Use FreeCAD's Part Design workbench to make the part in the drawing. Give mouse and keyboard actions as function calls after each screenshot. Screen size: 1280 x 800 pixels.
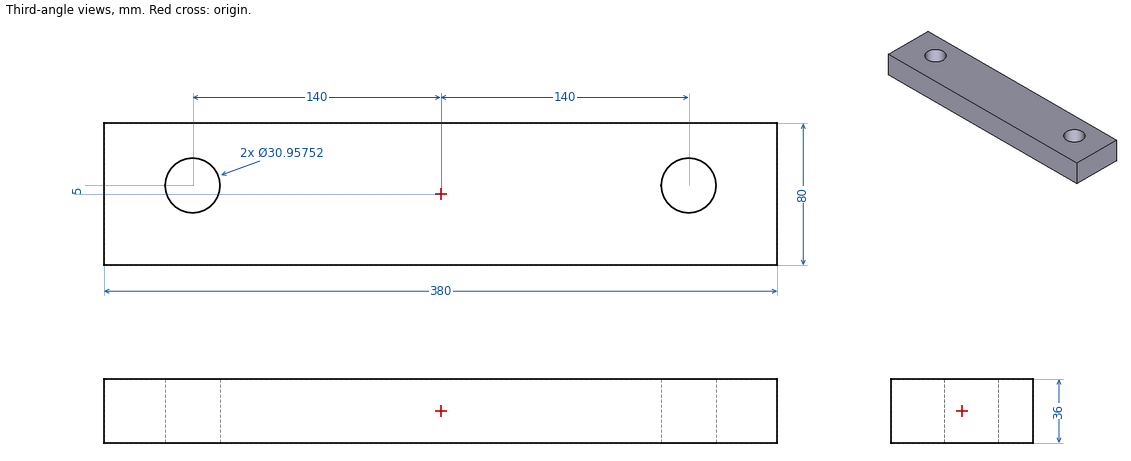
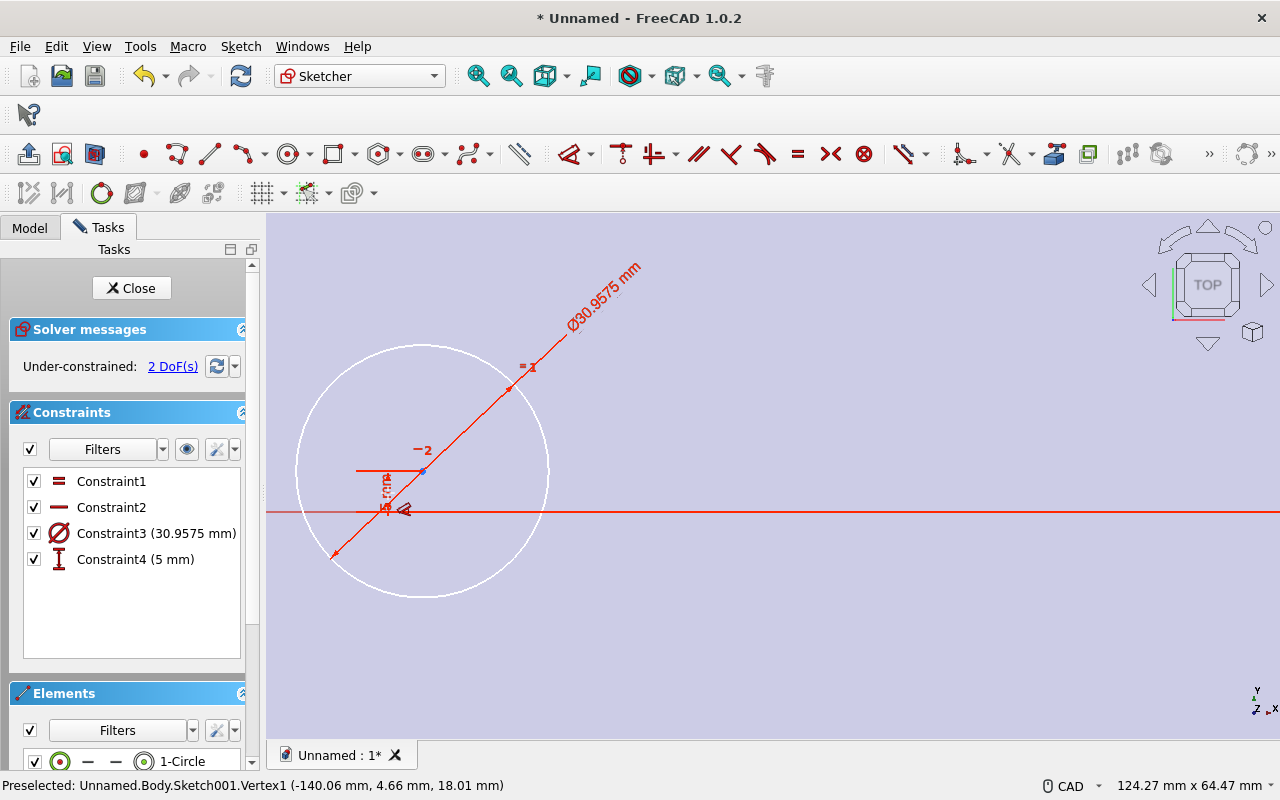
scroll(423, 478, down, 7)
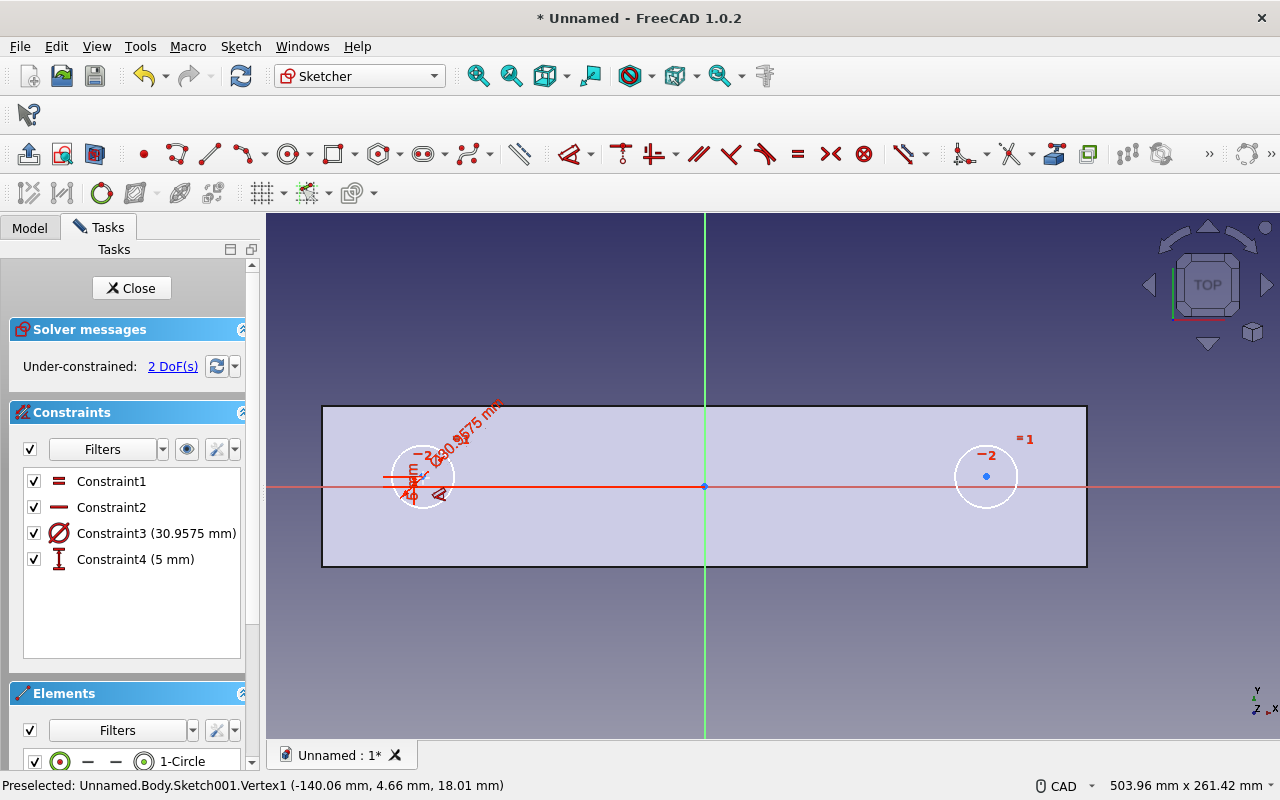
click(423, 477)
click(564, 521)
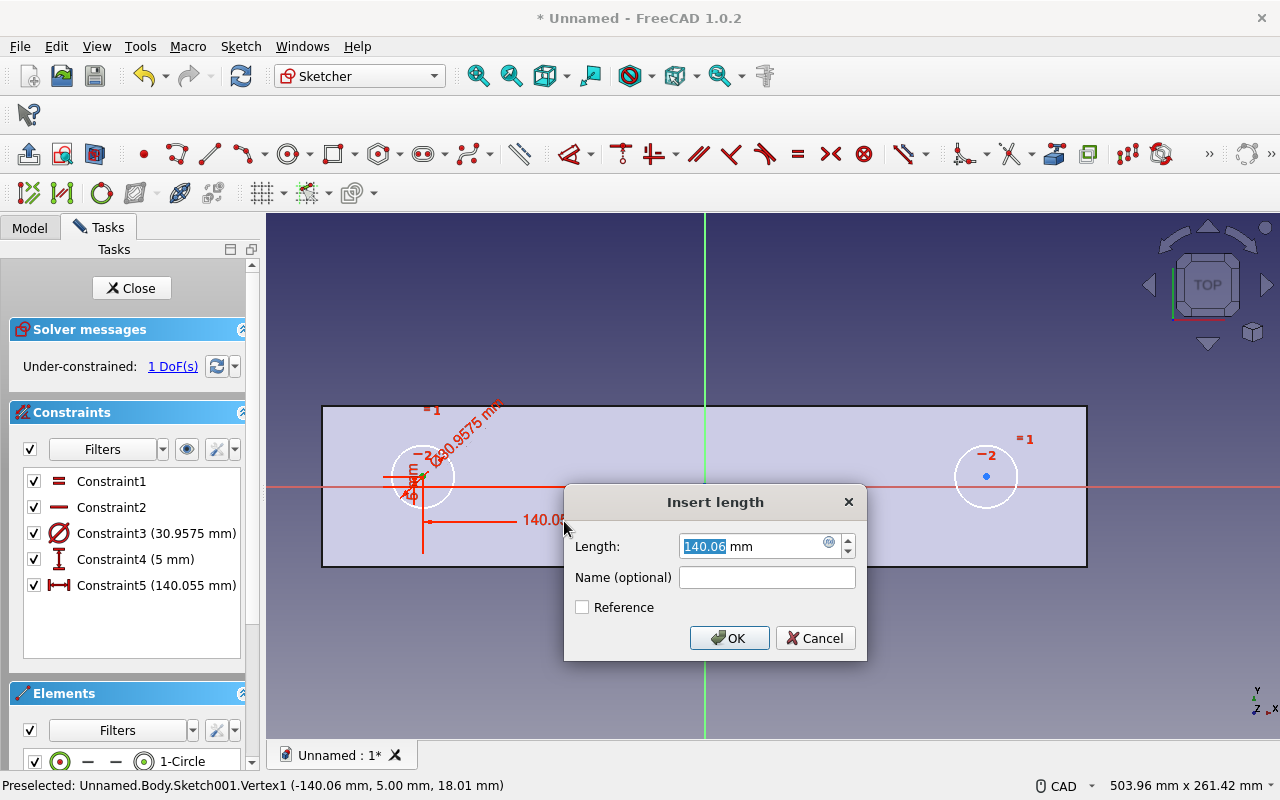
text(140)
key(Return)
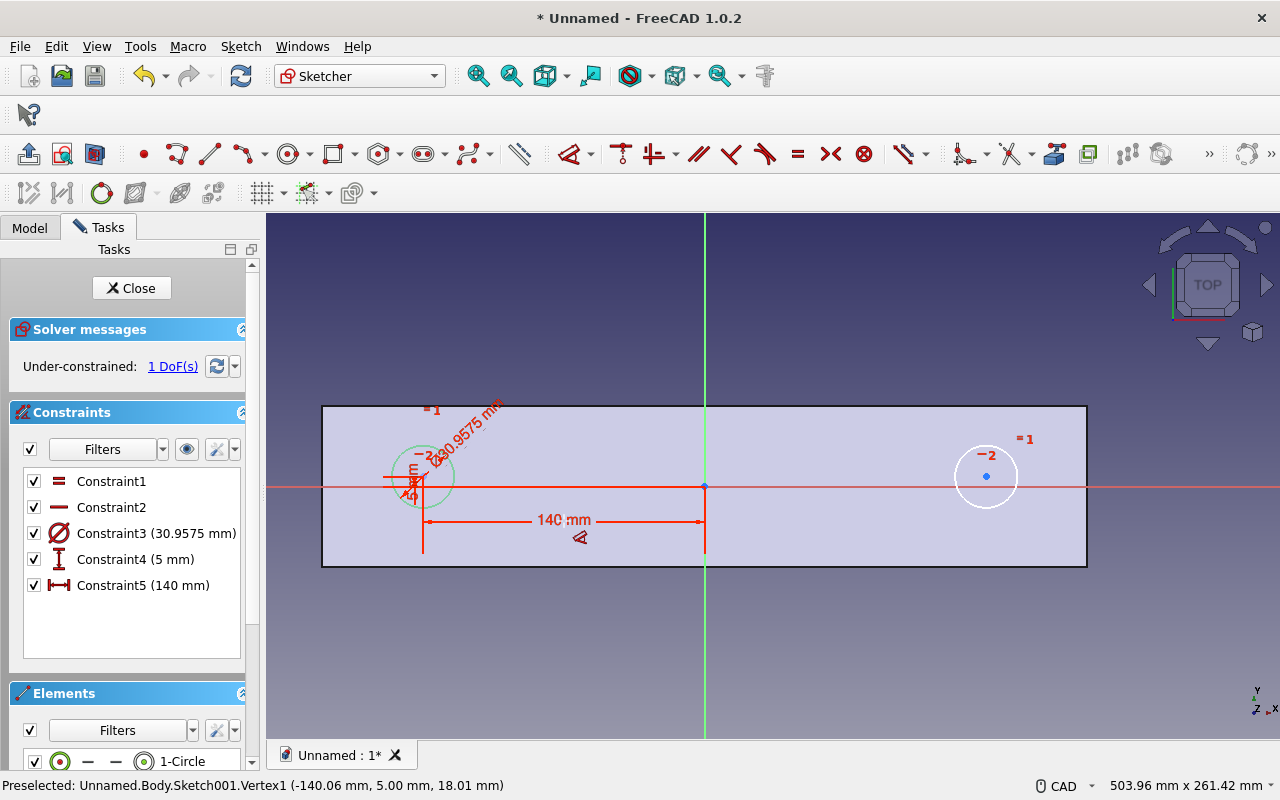
click(986, 477)
click(846, 521)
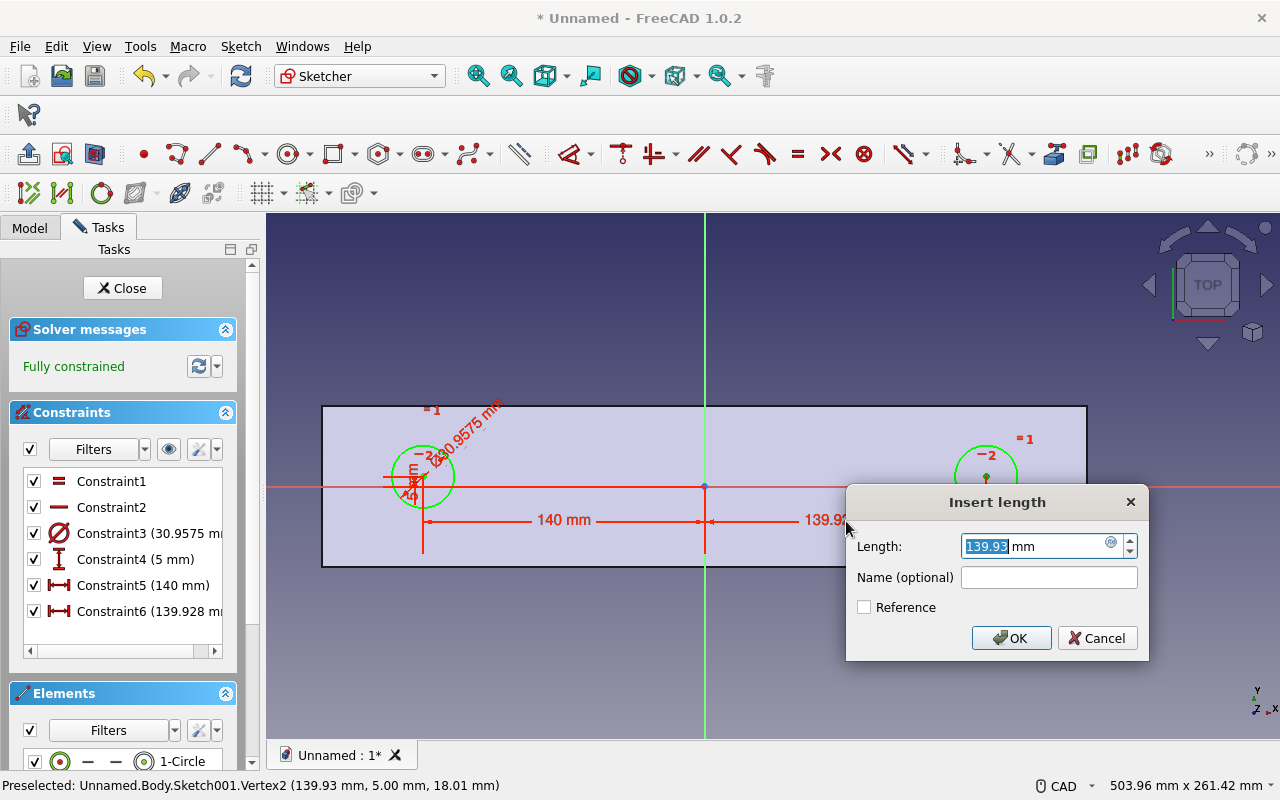
text(140)
key(Return)
key(Escape)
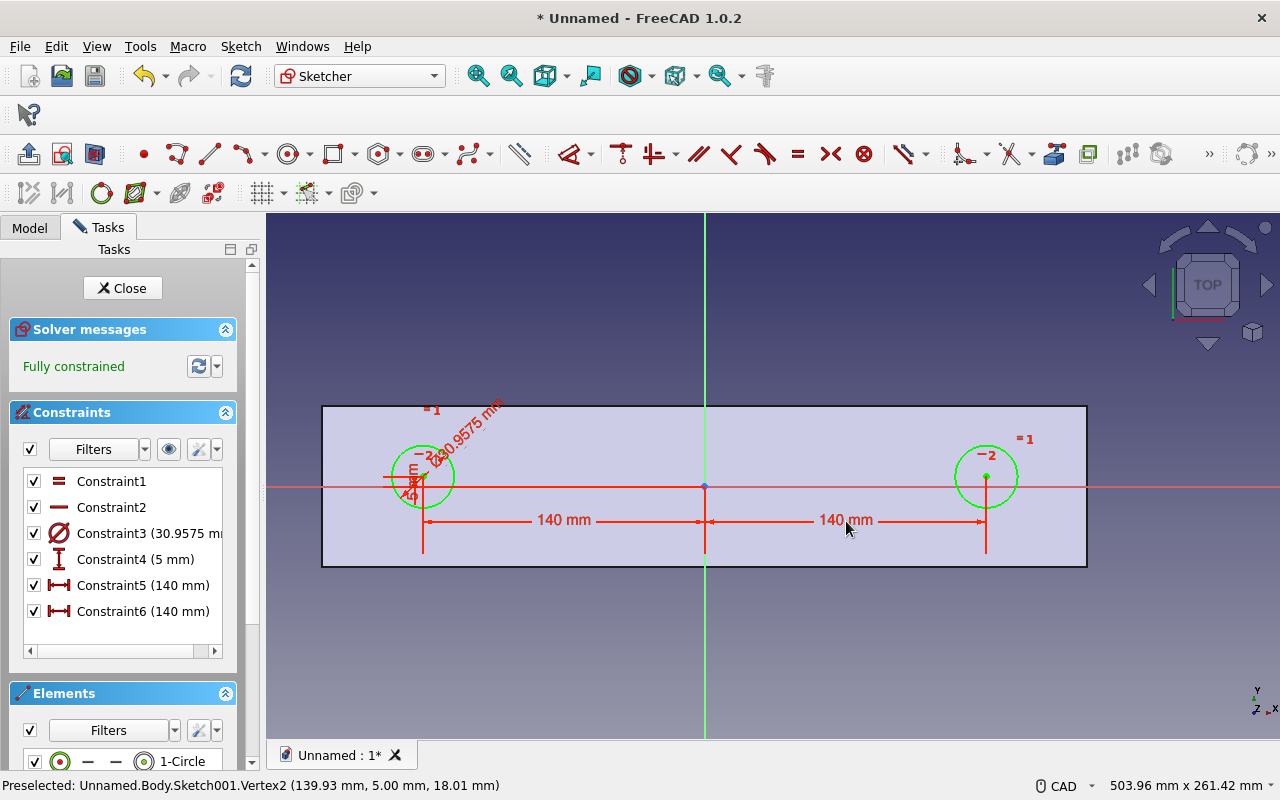
click(123, 288)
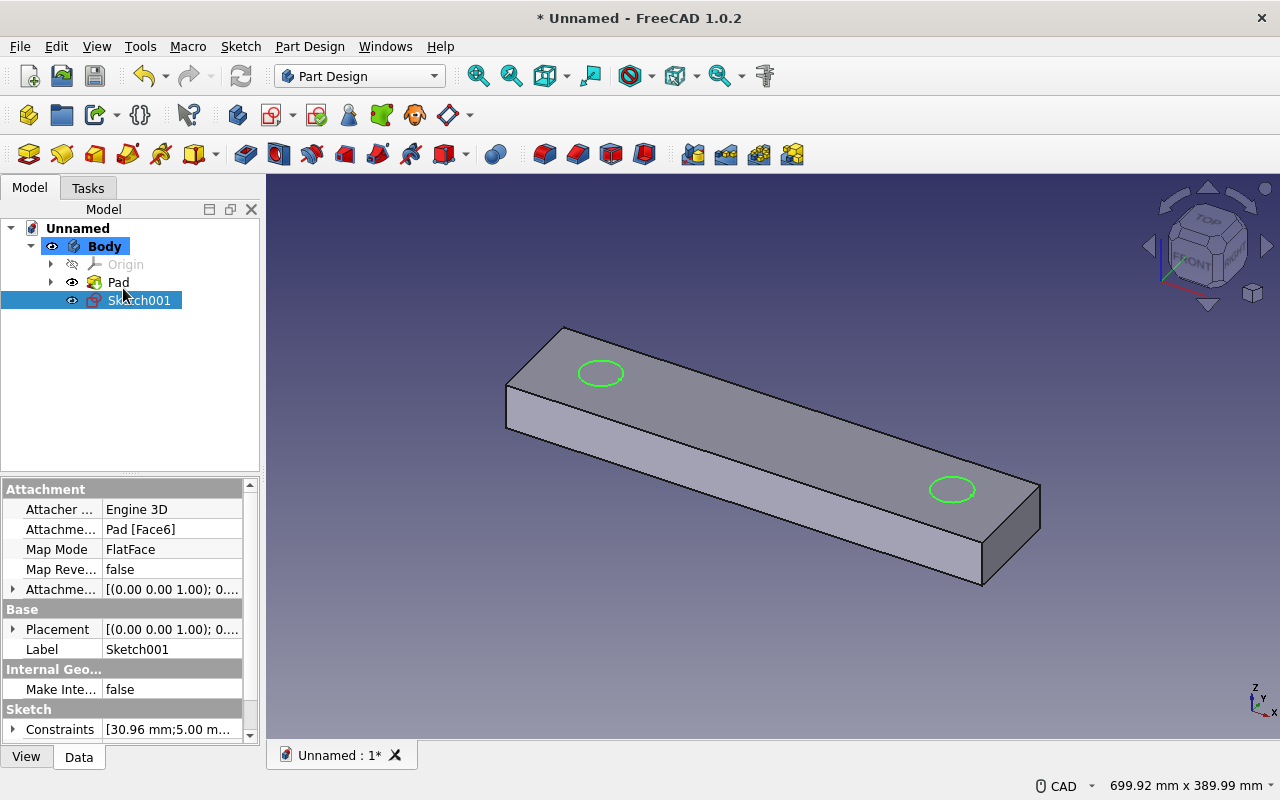
click(246, 154)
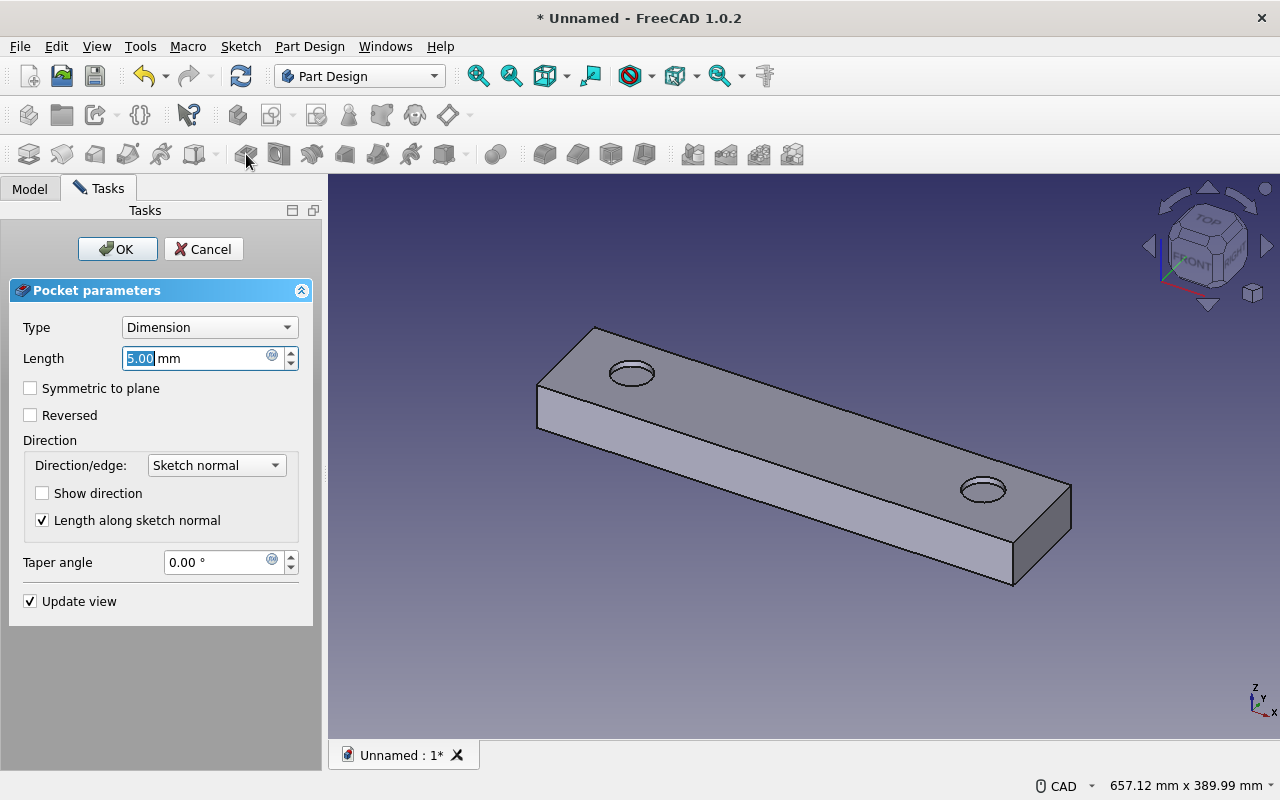
click(210, 328)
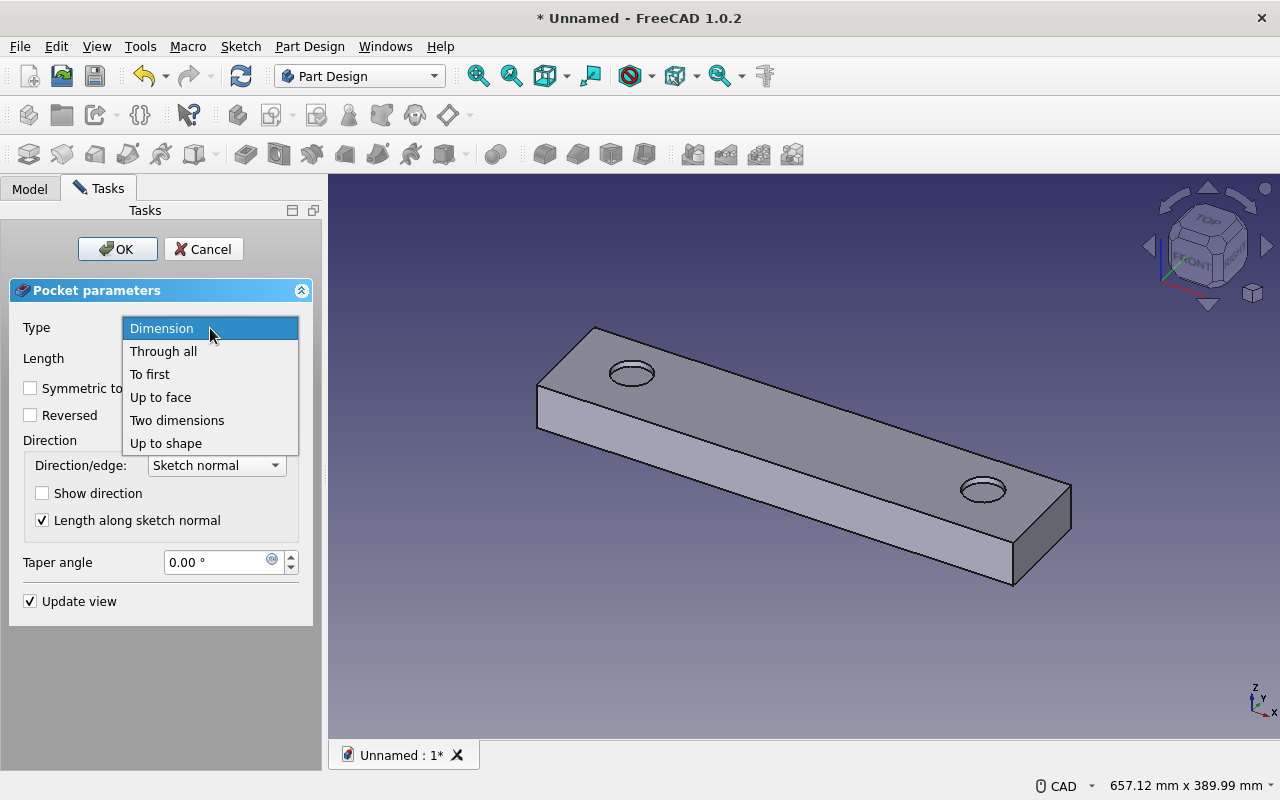
click(208, 352)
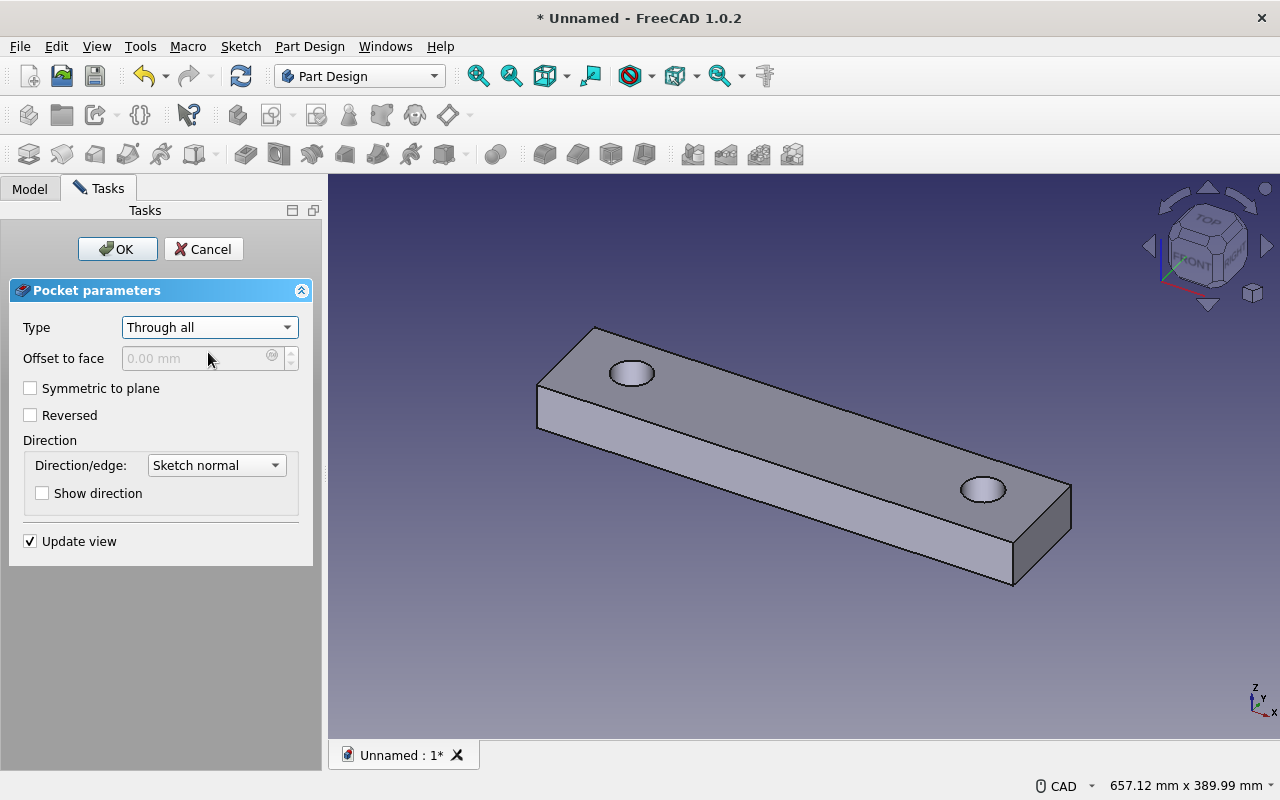
click(118, 249)